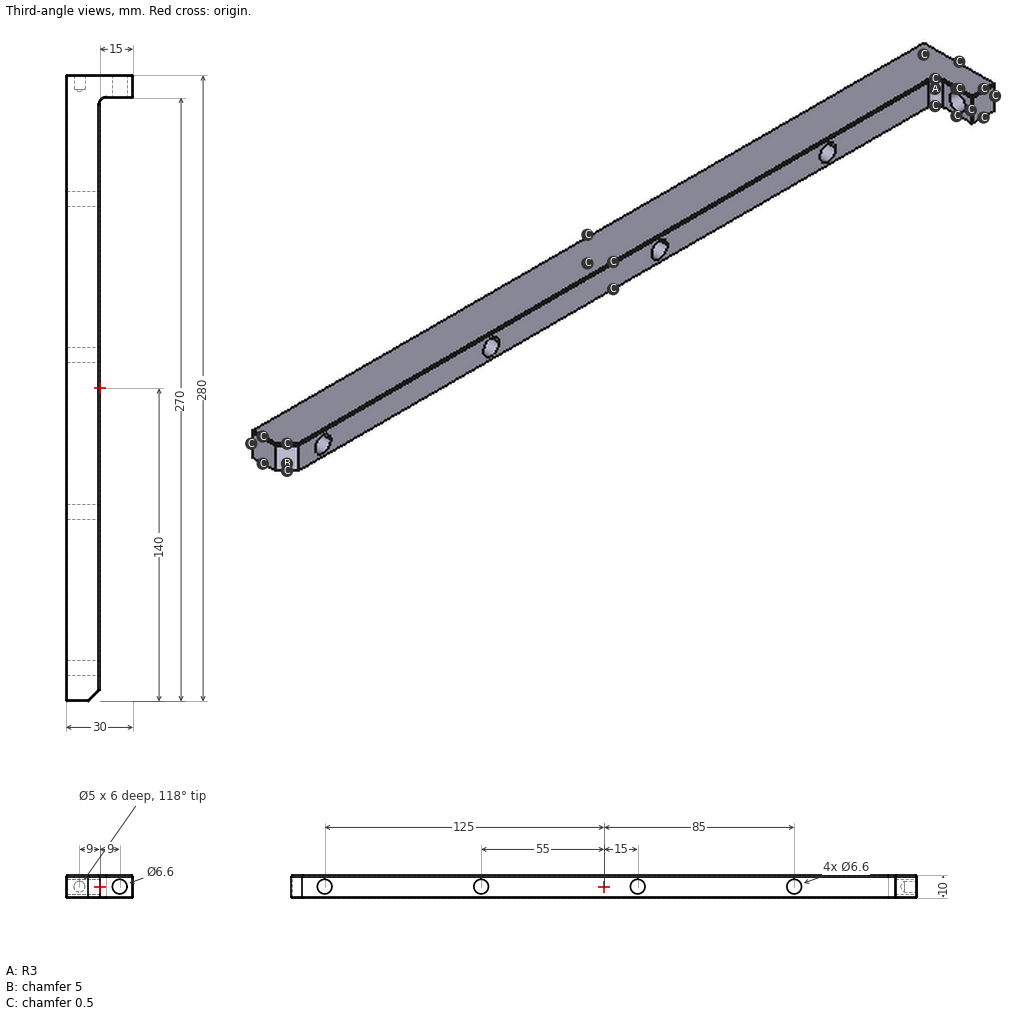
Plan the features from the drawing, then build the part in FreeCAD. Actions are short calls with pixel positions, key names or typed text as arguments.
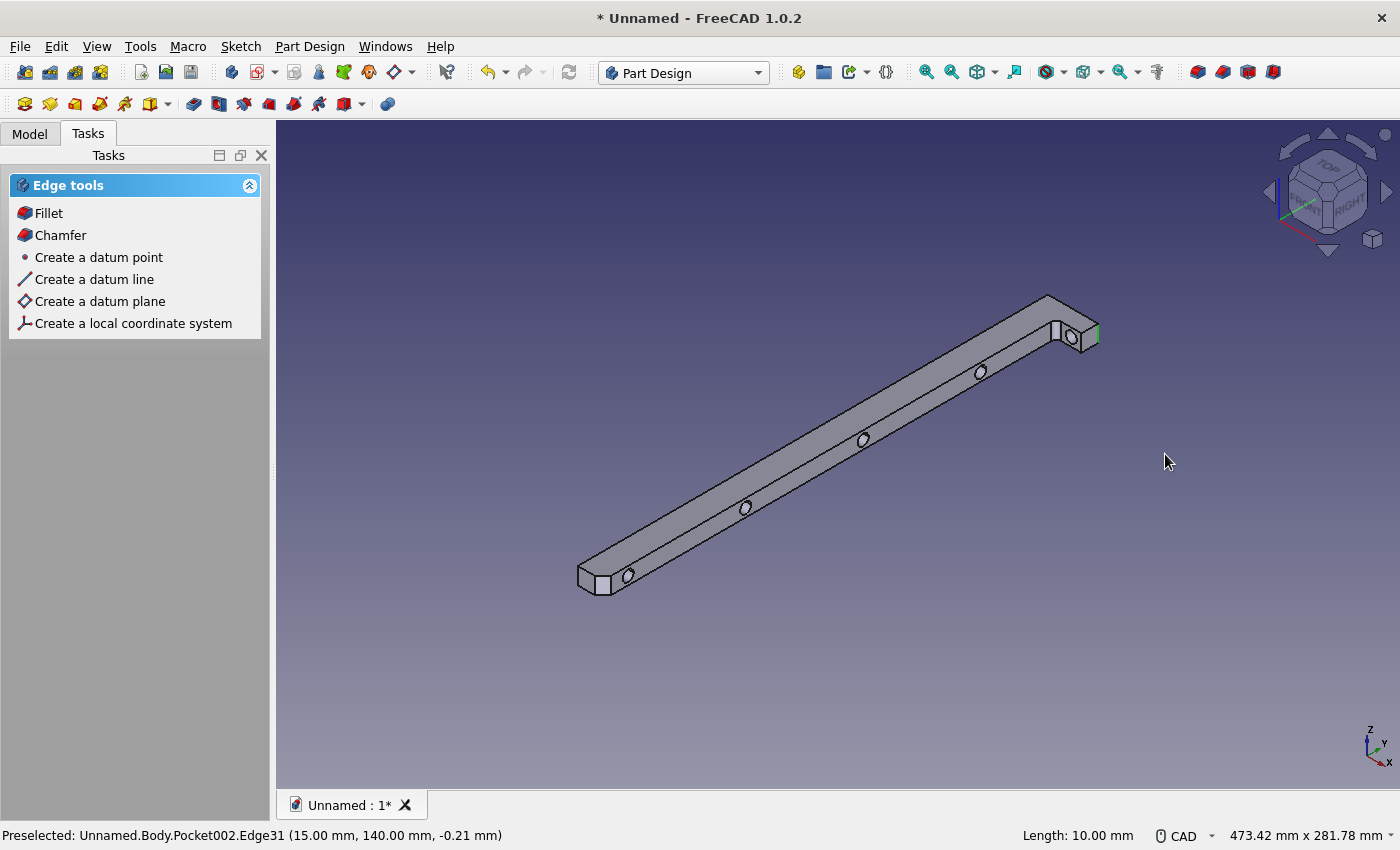
click(1025, 319, ctrl)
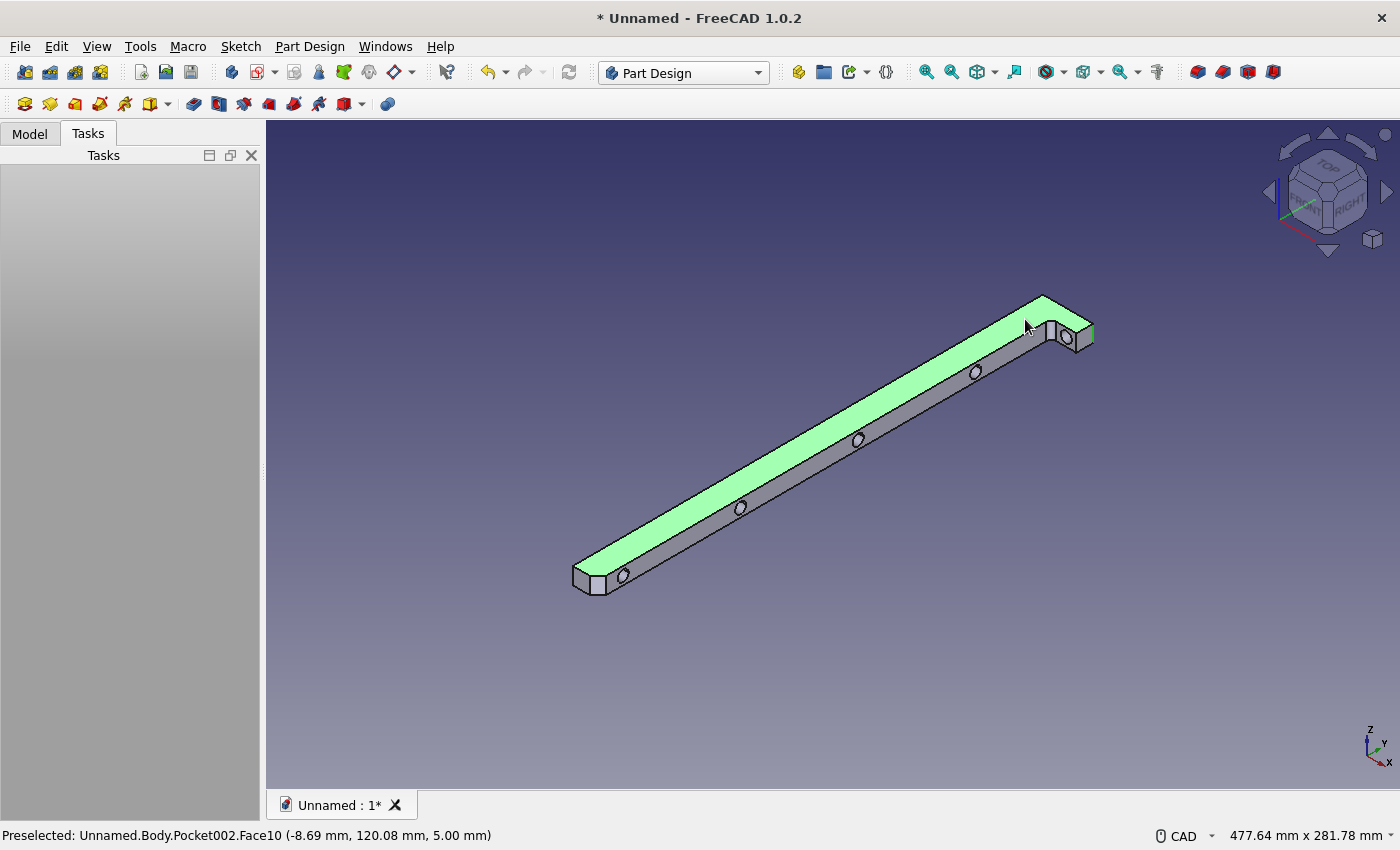
click(1076, 342, ctrl)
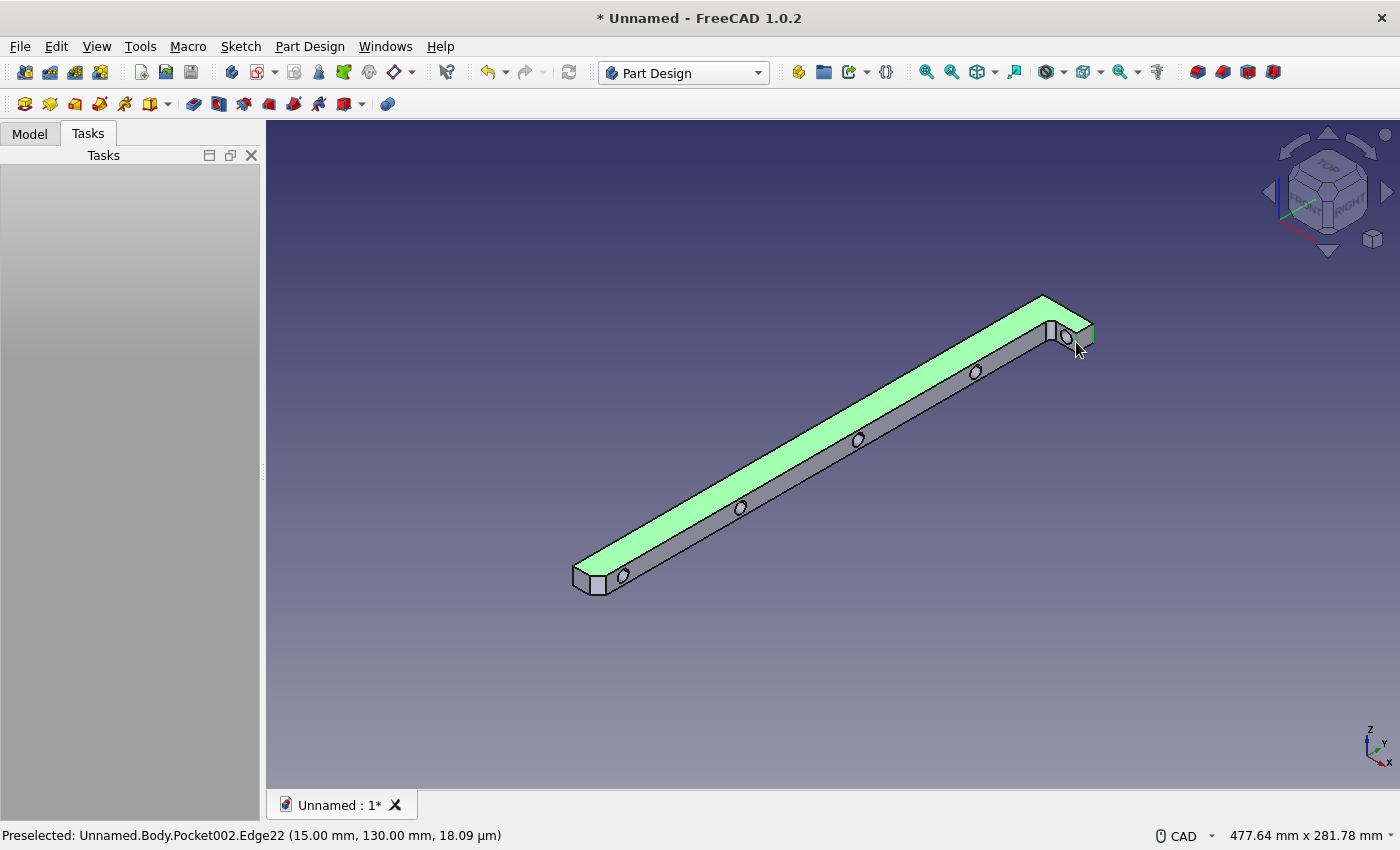
key(2)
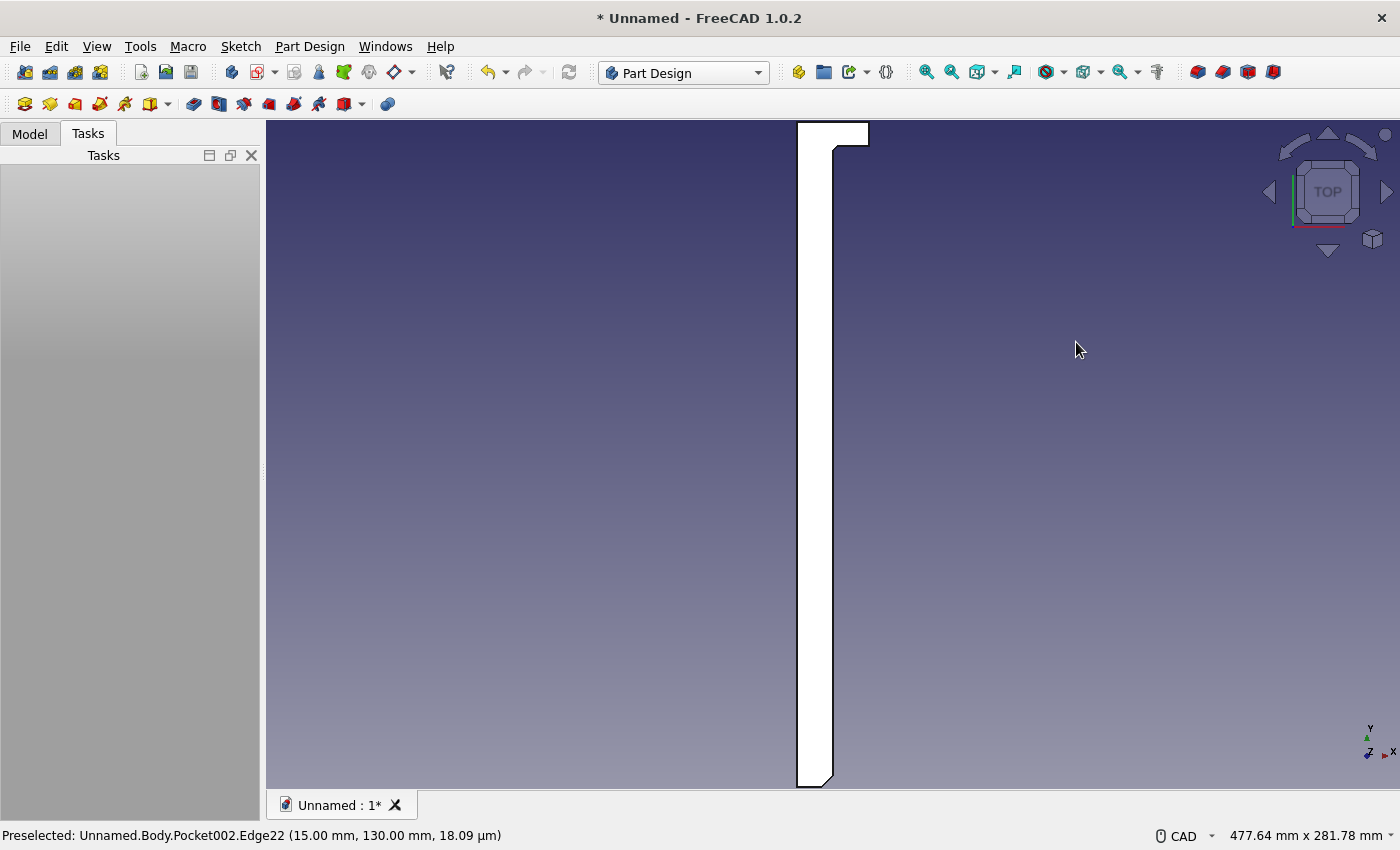
key(1)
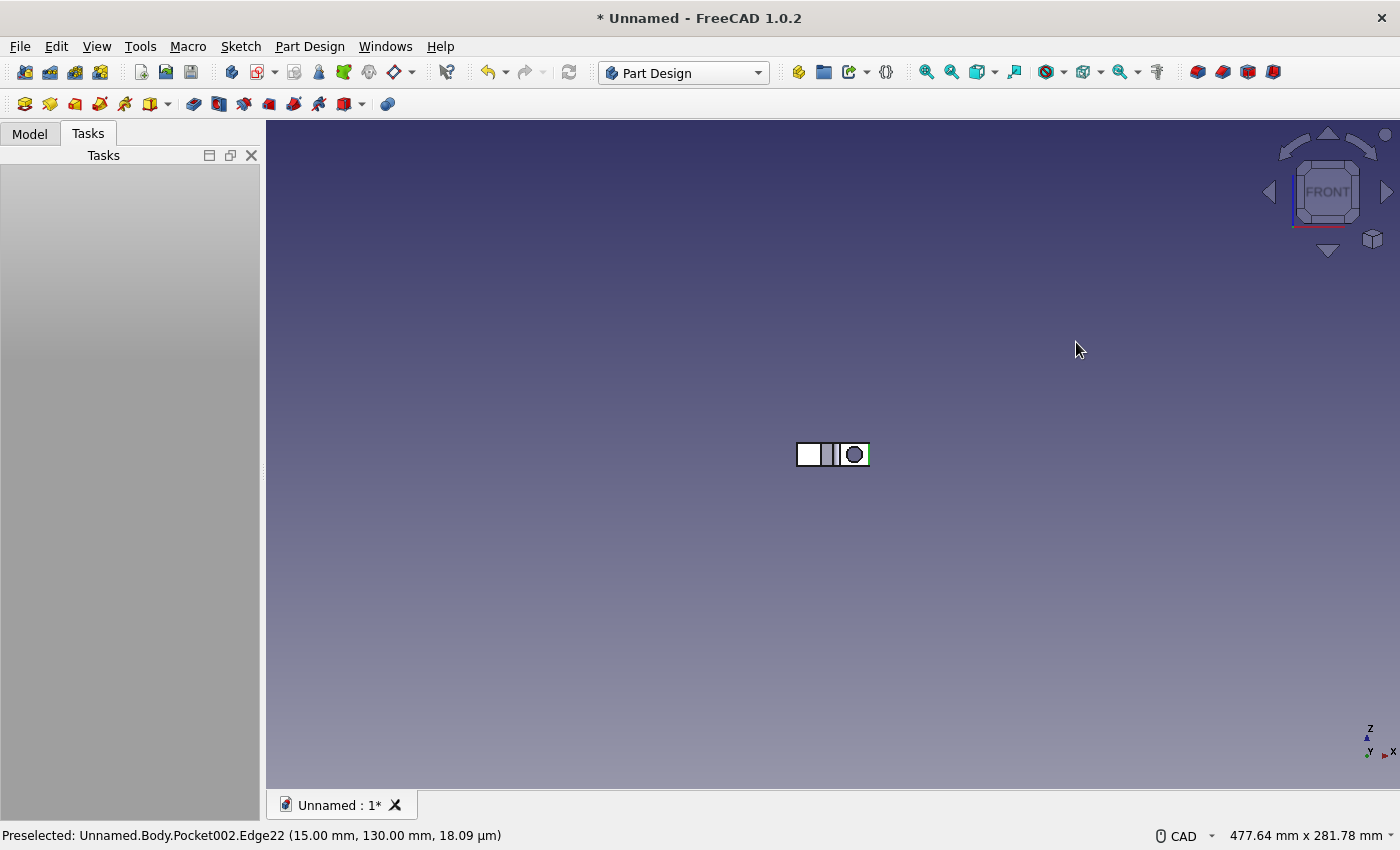
key(v)
key(f)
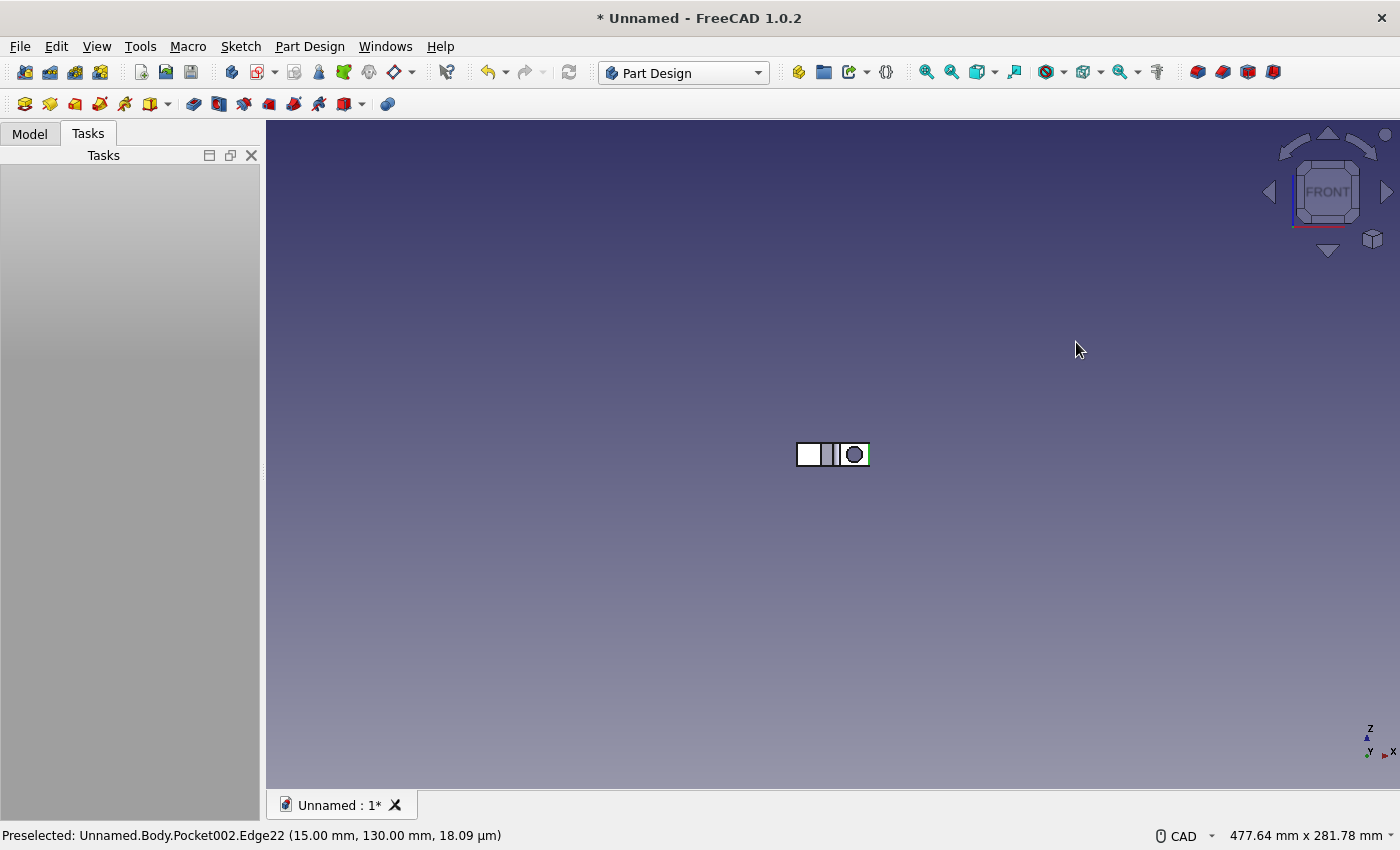
click(797, 454, ctrl)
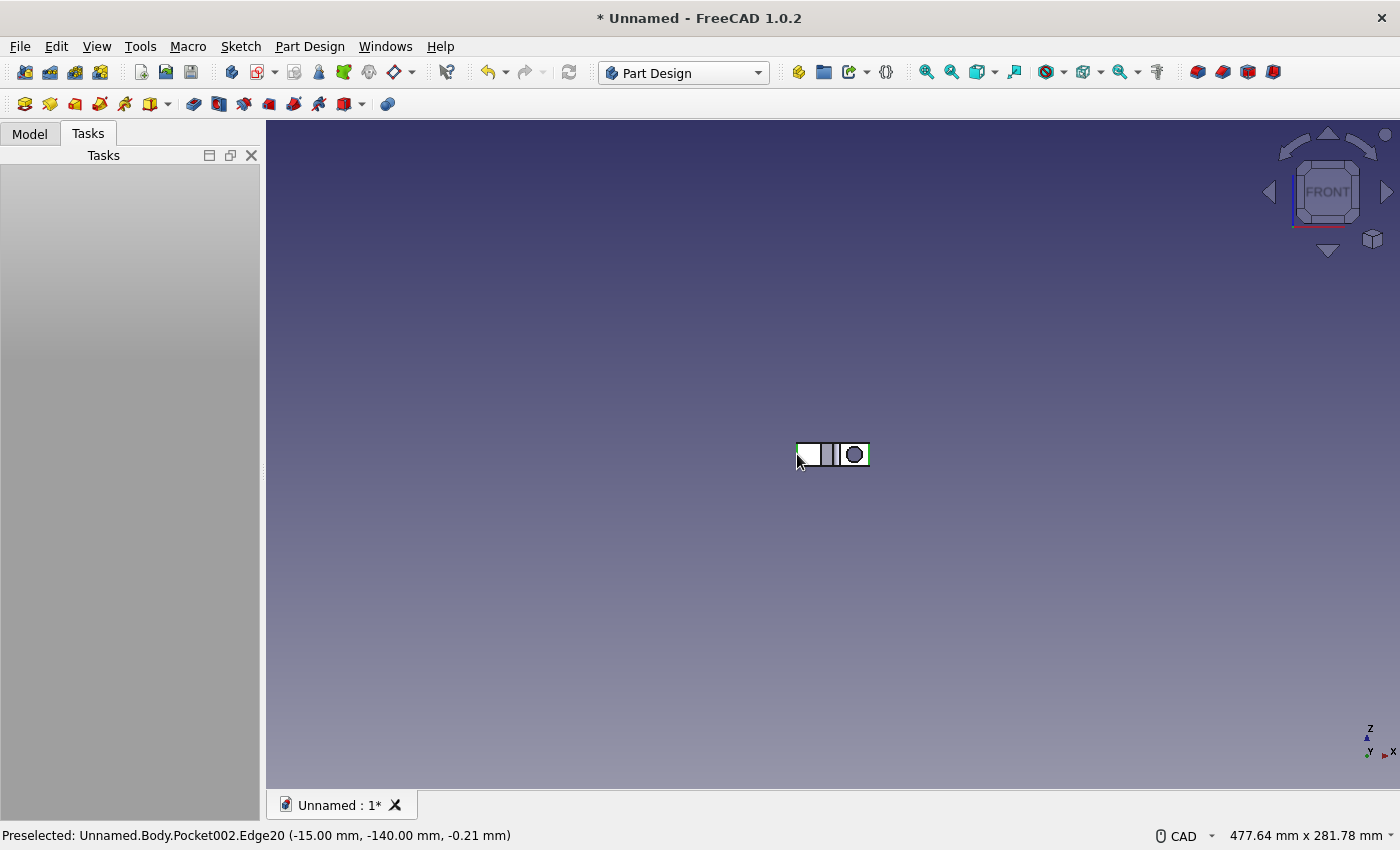
key(3)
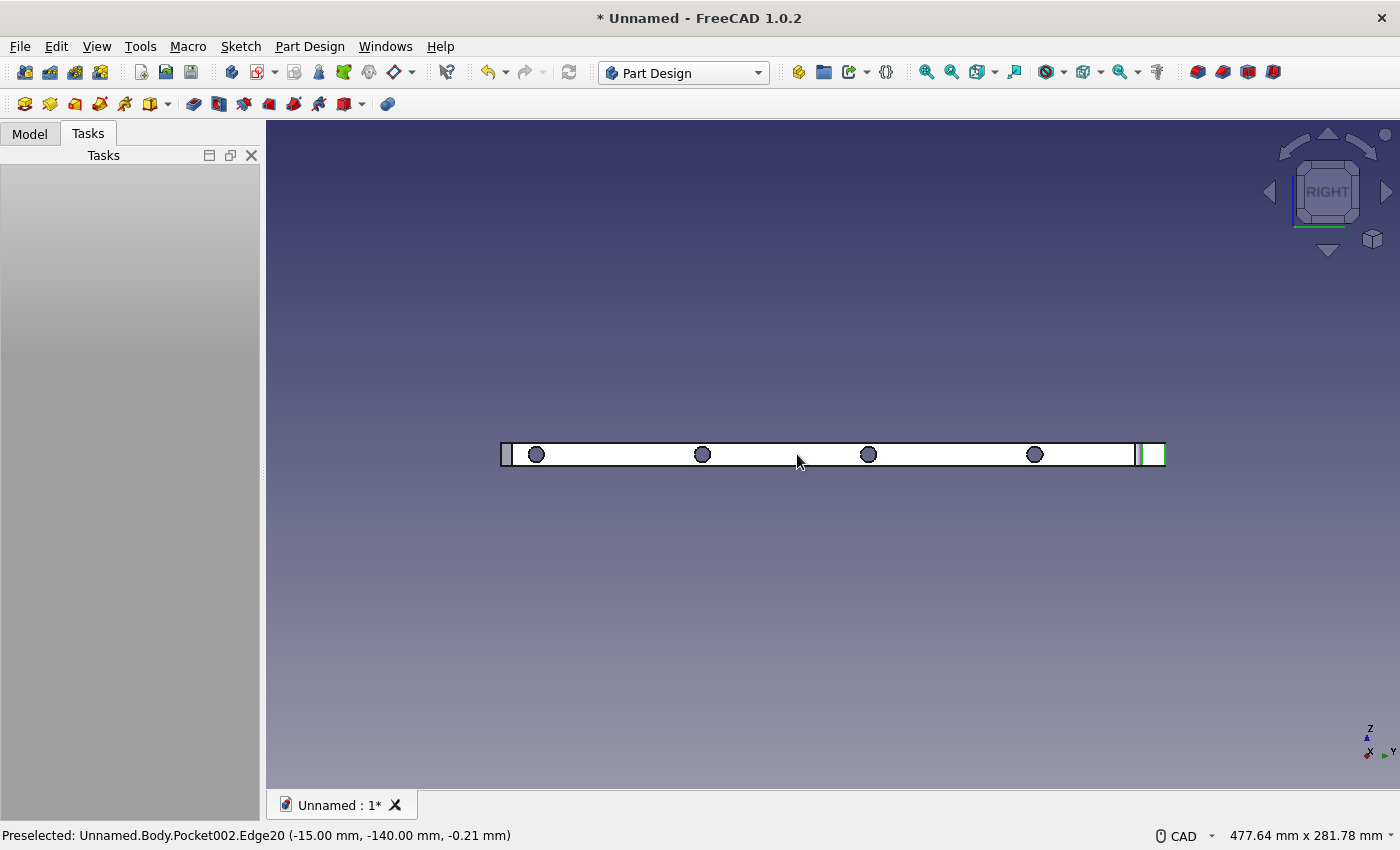
key(5)